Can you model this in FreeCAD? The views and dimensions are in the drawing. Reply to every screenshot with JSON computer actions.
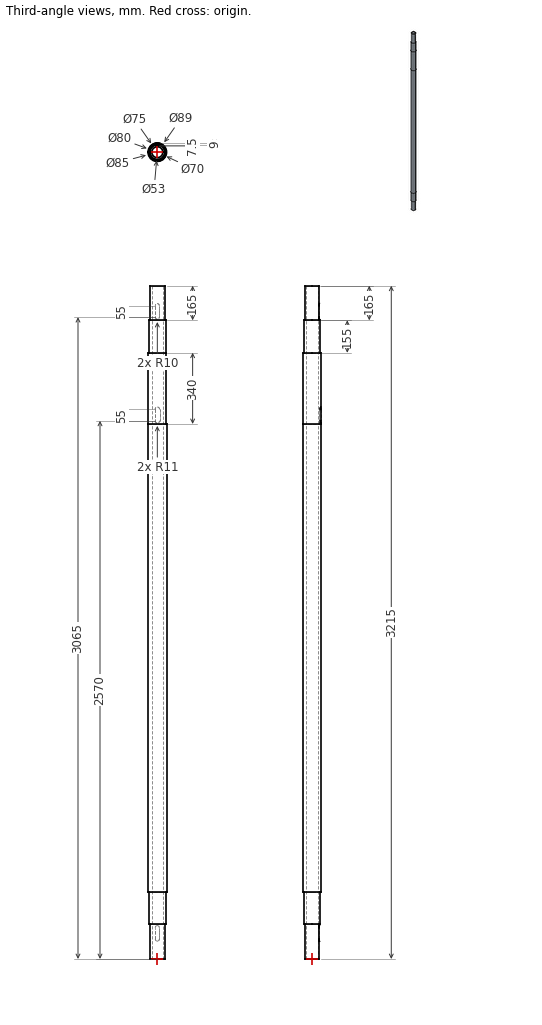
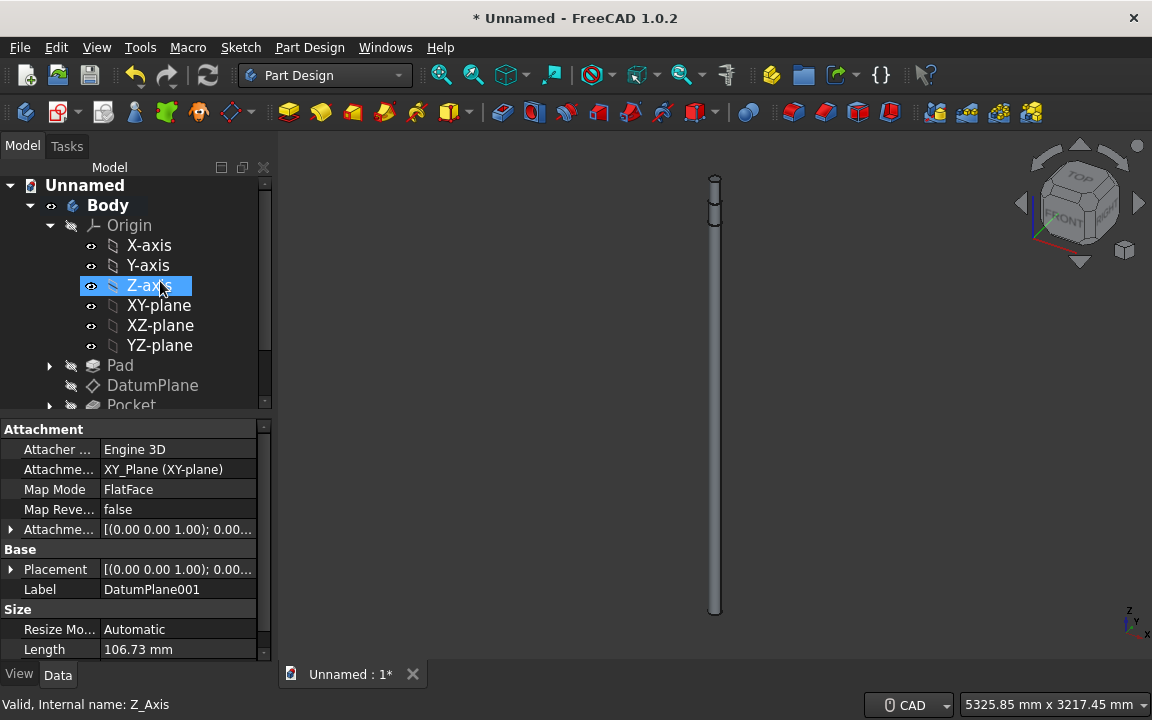
{"action": "left_click", "coordinate": [136, 306]}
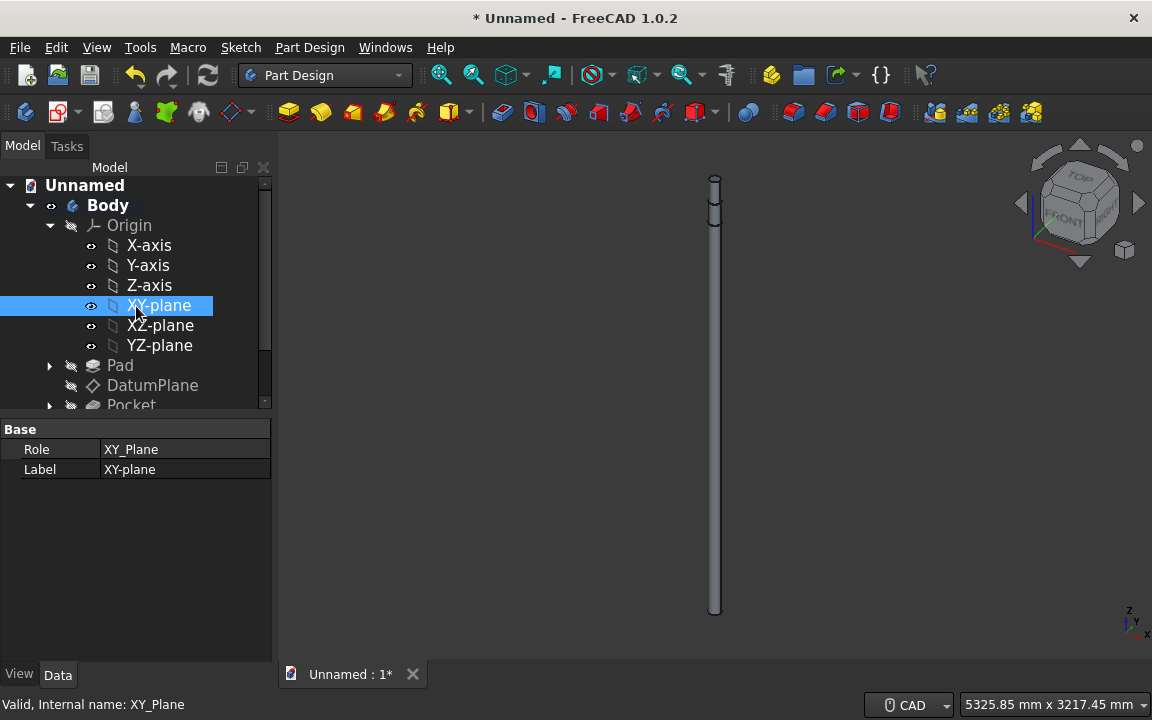
{"action": "left_click", "coordinate": [232, 112]}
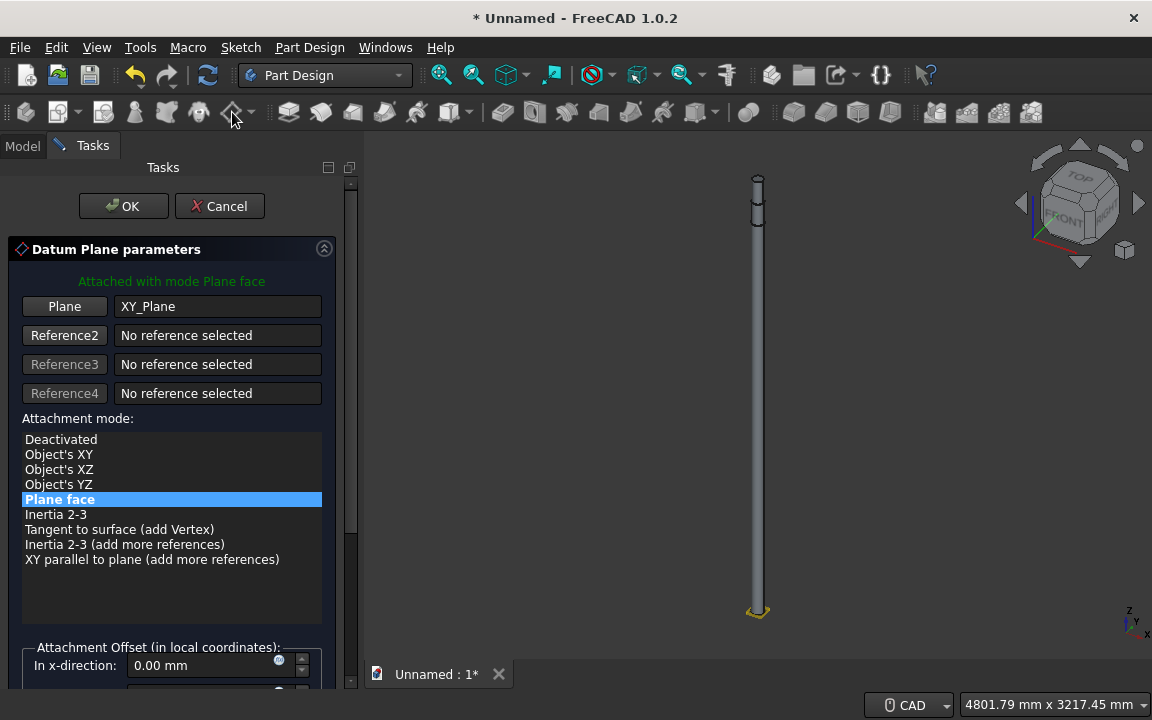
{"action": "scroll", "coordinate": [351, 432], "scroll_direction": "down", "scroll_amount": 2}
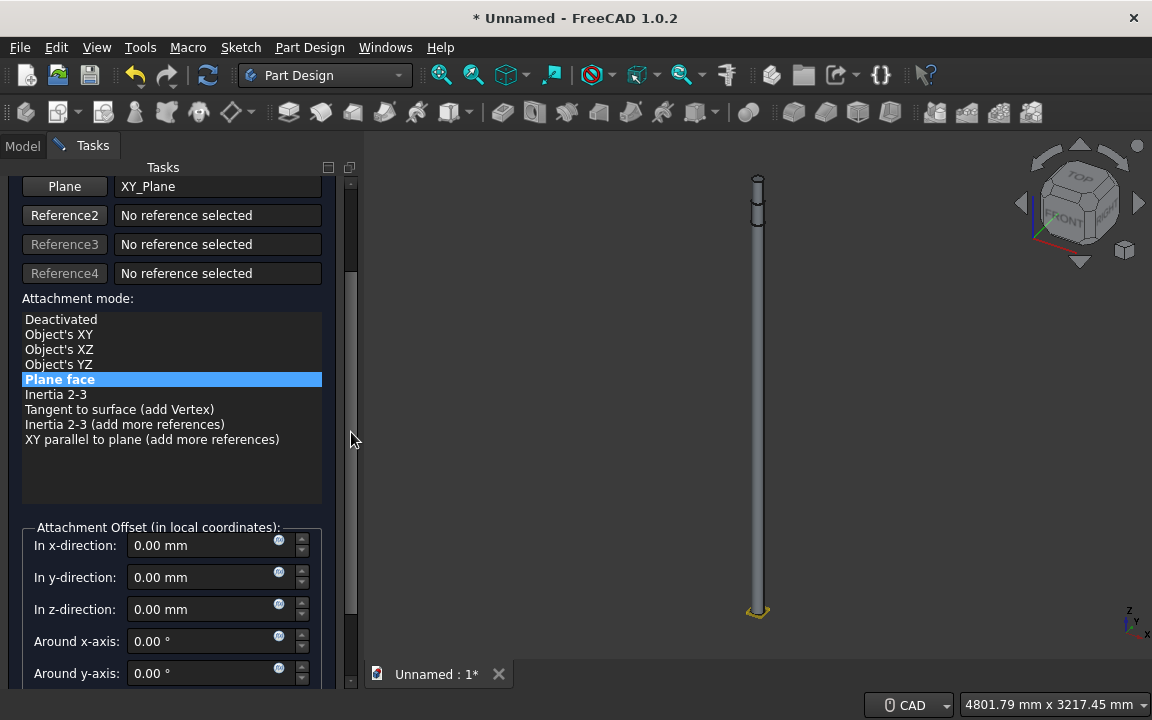
{"action": "triple_click", "coordinate": [210, 609]}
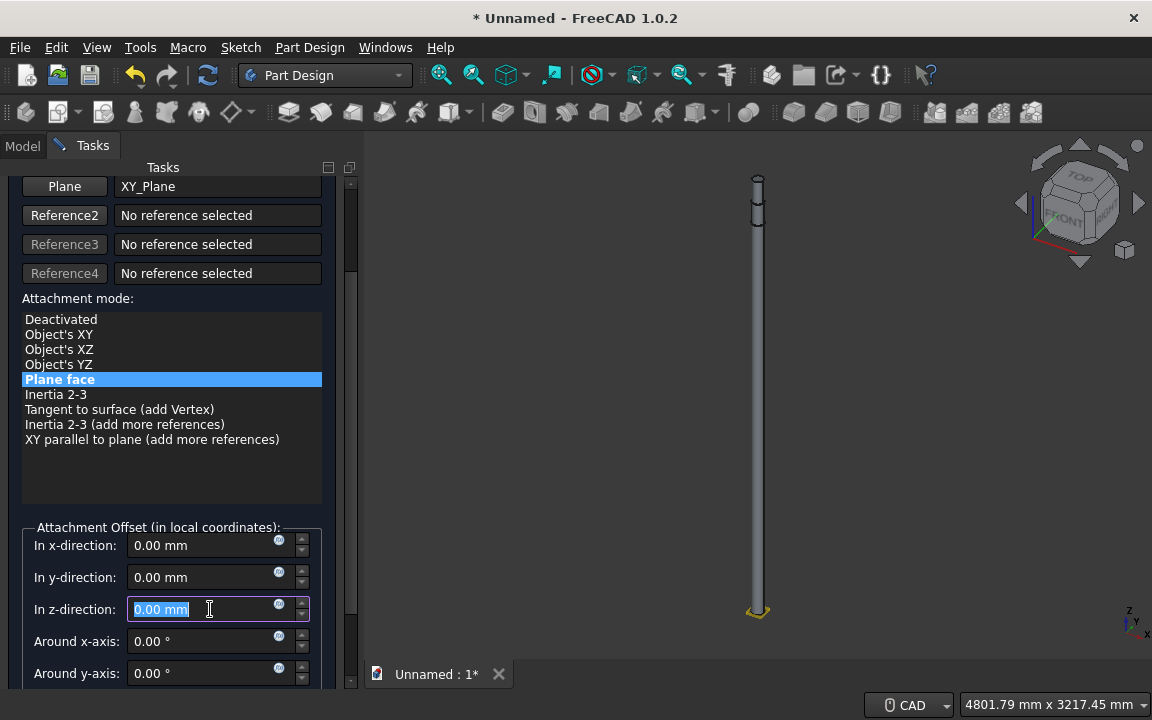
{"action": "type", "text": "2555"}
{"action": "key", "text": "Tab"}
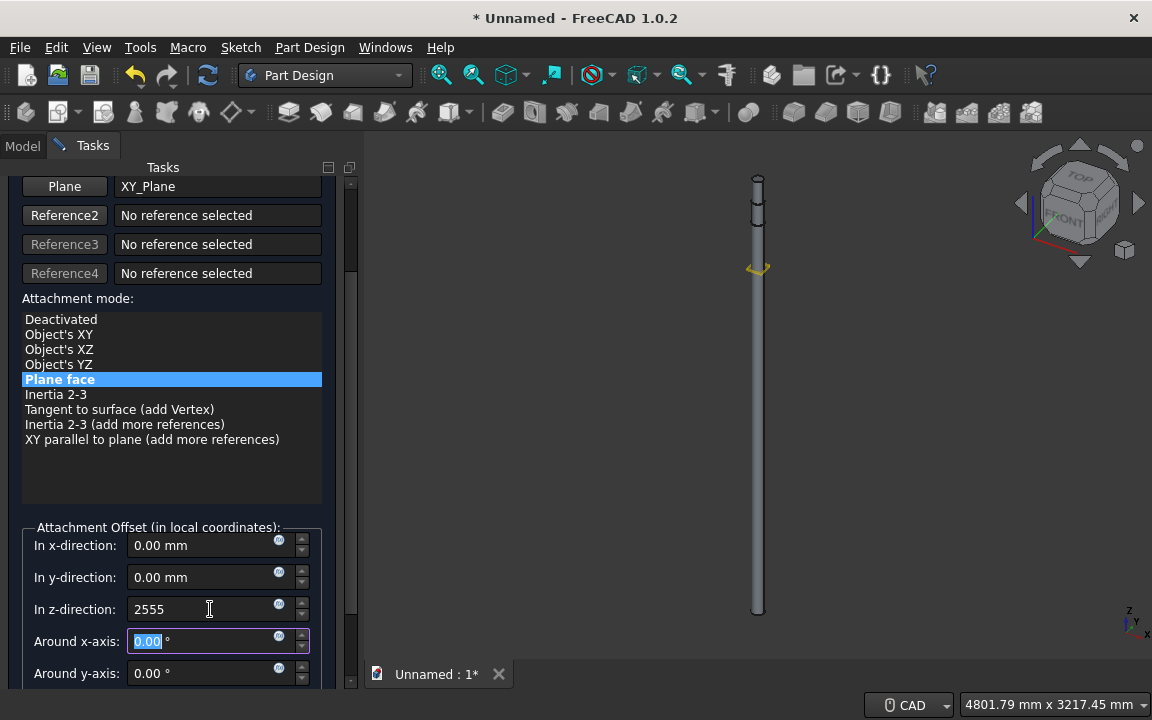
{"action": "scroll", "coordinate": [351, 432], "scroll_direction": "up", "scroll_amount": 3}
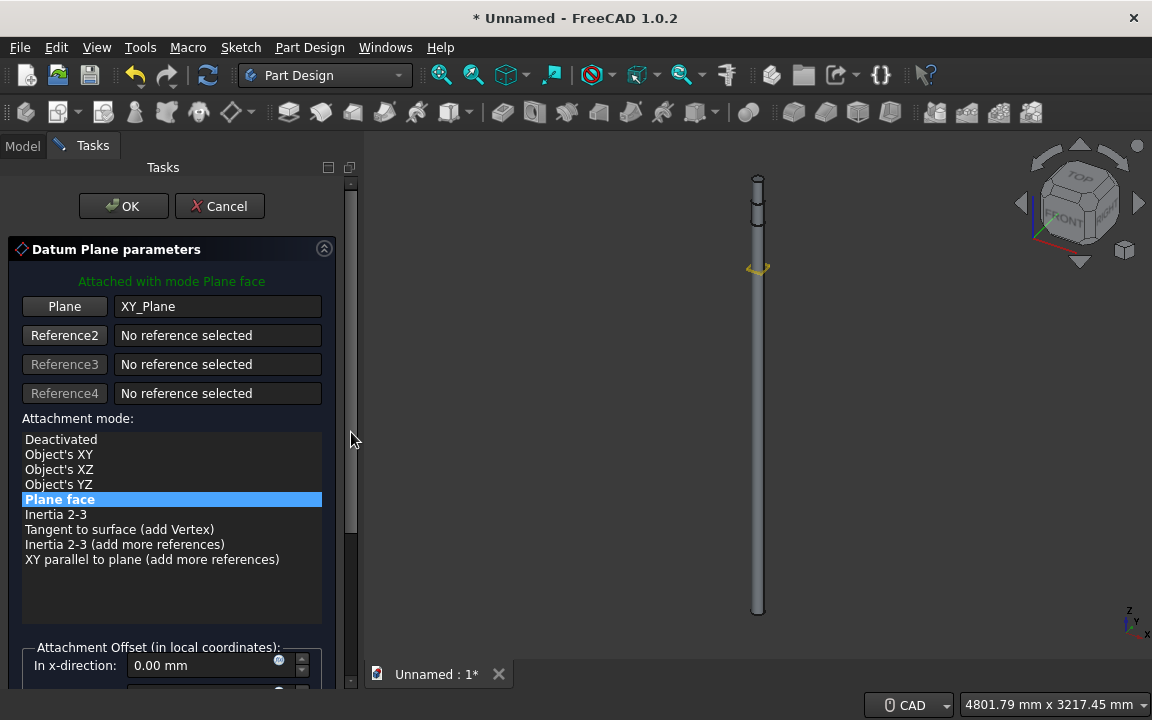
{"action": "left_click", "coordinate": [124, 206]}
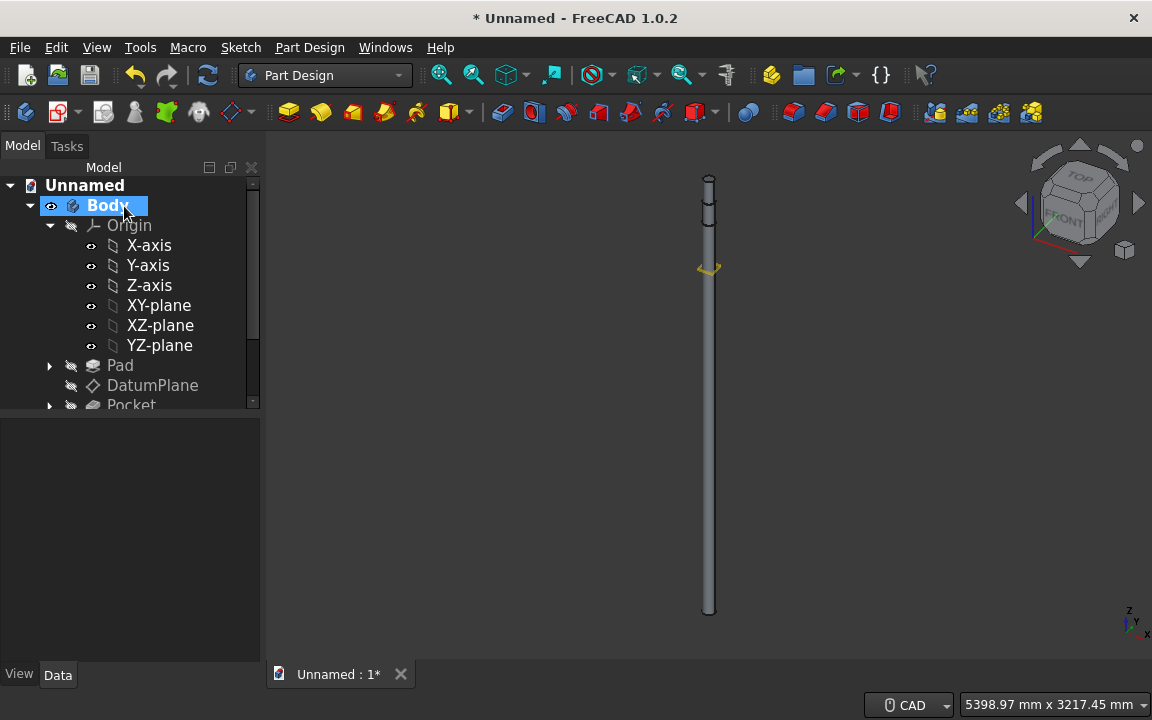
{"action": "scroll", "coordinate": [100, 301], "scroll_direction": "down", "scroll_amount": 3}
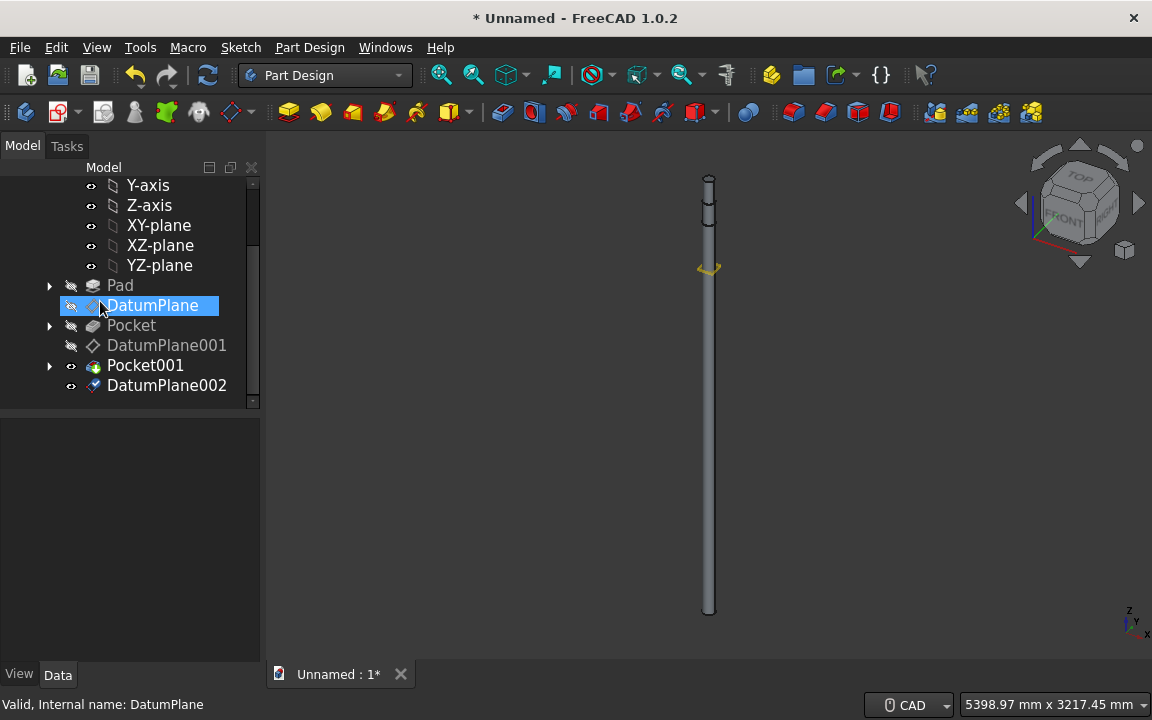
{"action": "left_click", "coordinate": [116, 386]}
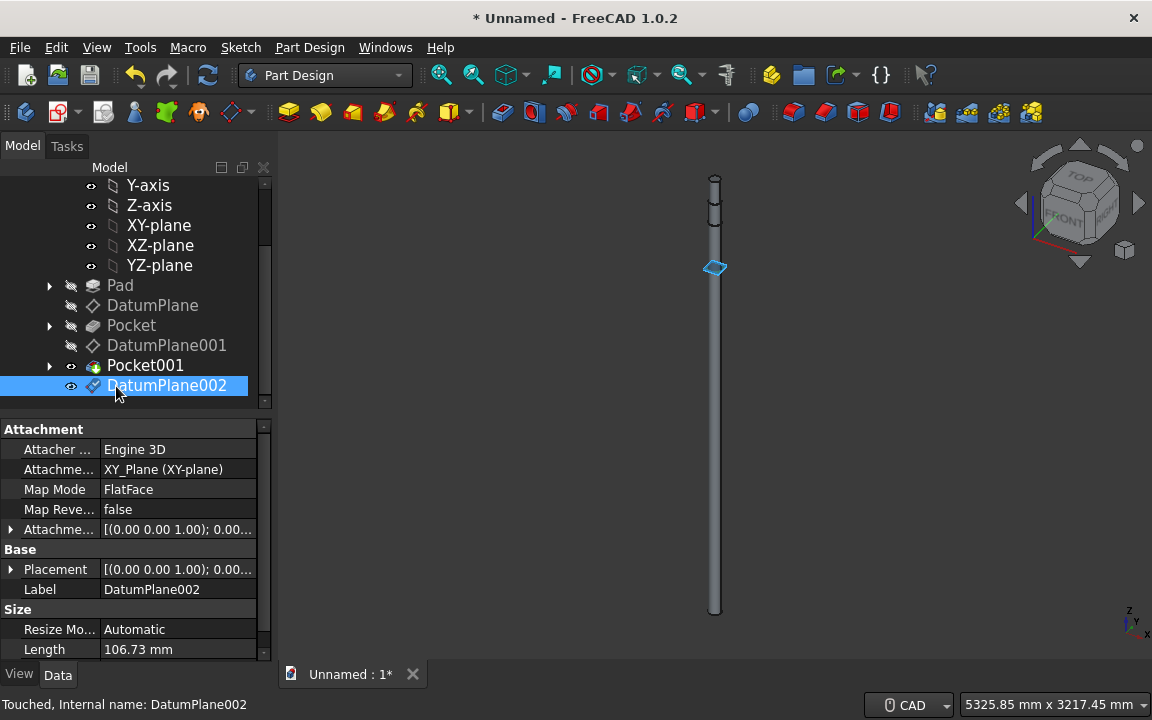
{"action": "left_click", "coordinate": [58, 112]}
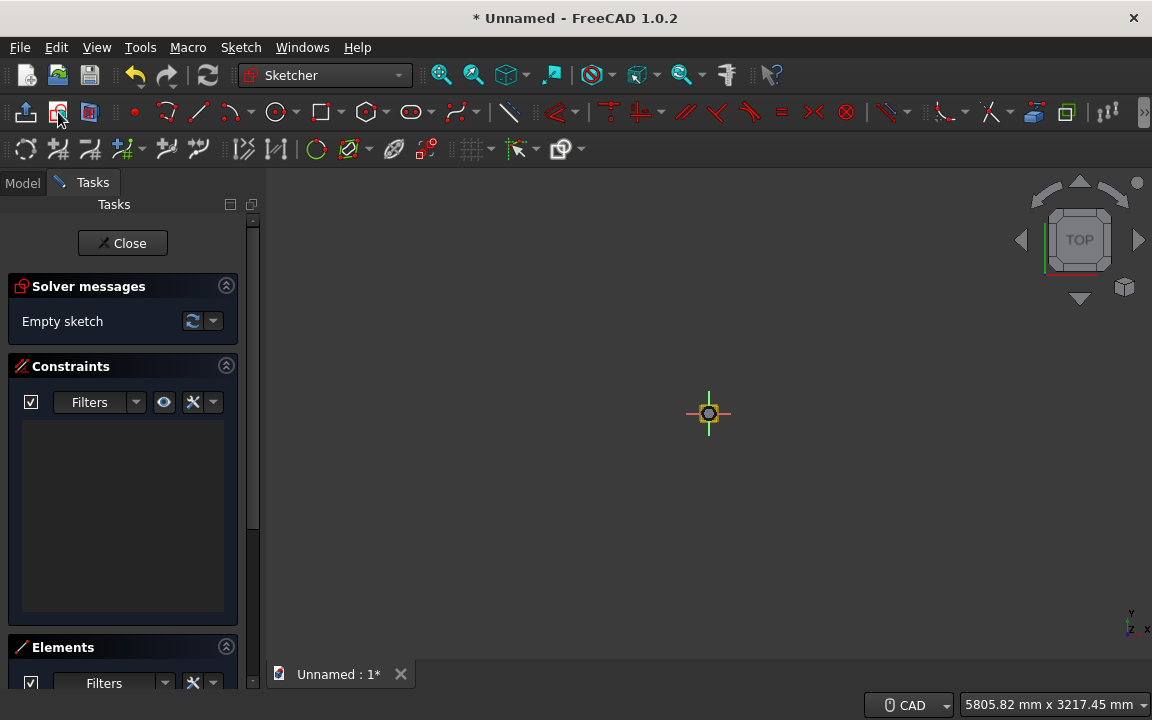
{"action": "left_click", "coordinate": [90, 112]}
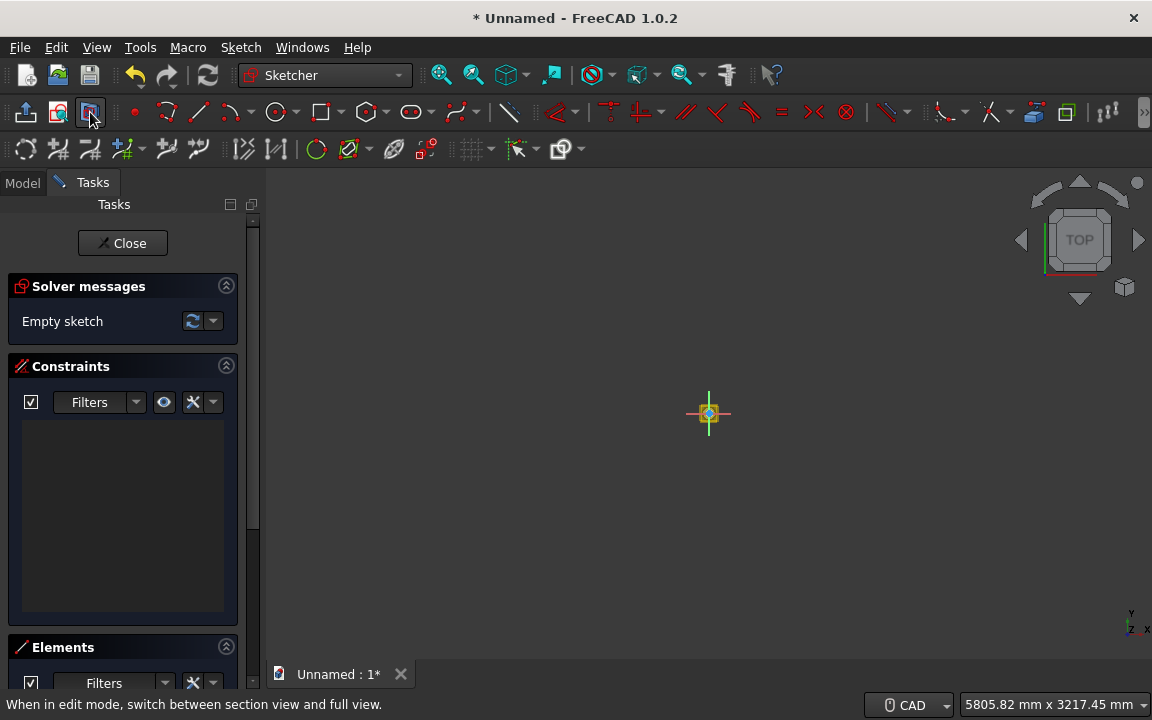
{"action": "scroll", "coordinate": [713, 414], "scroll_direction": "up", "scroll_amount": 15}